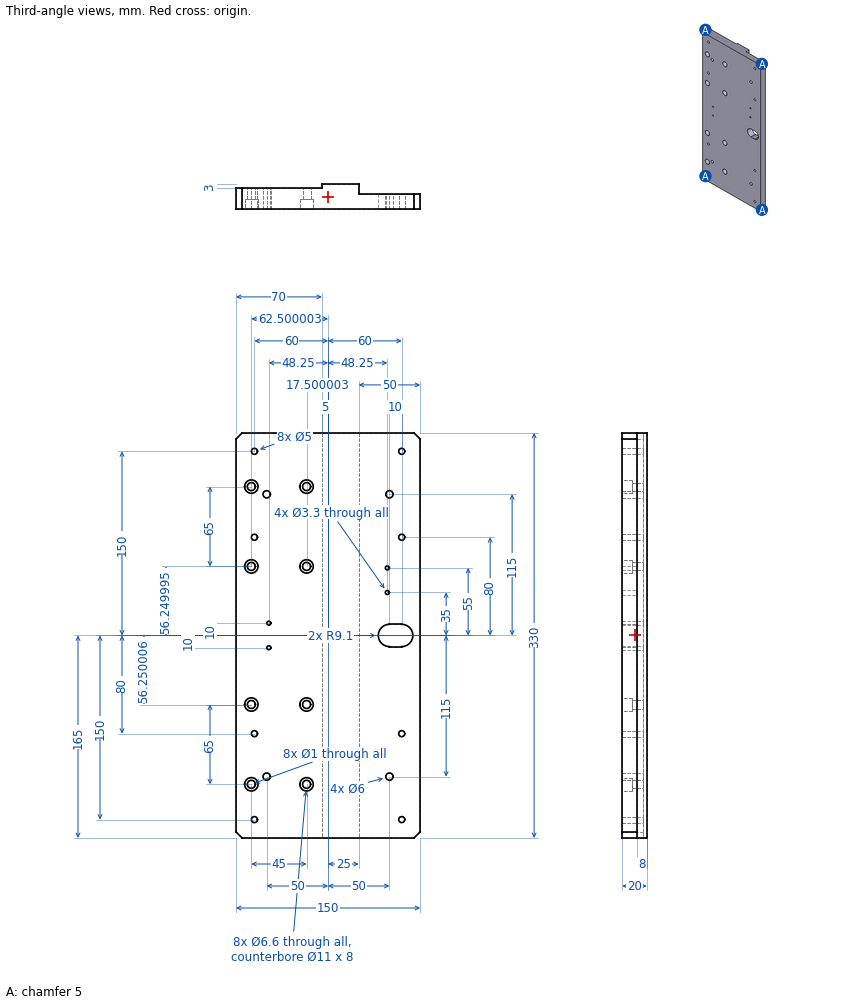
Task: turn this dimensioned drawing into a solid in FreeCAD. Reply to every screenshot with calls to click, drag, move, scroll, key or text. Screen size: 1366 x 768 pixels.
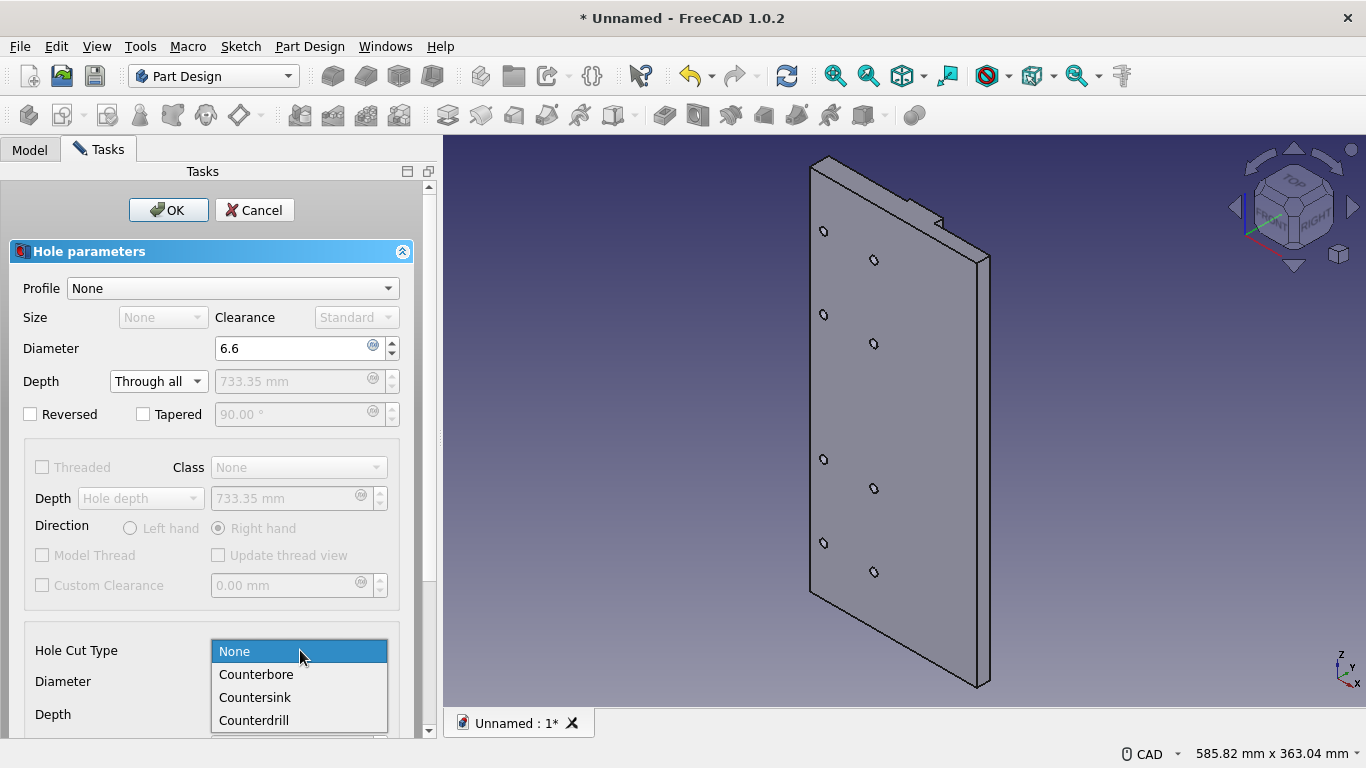
click(298, 674)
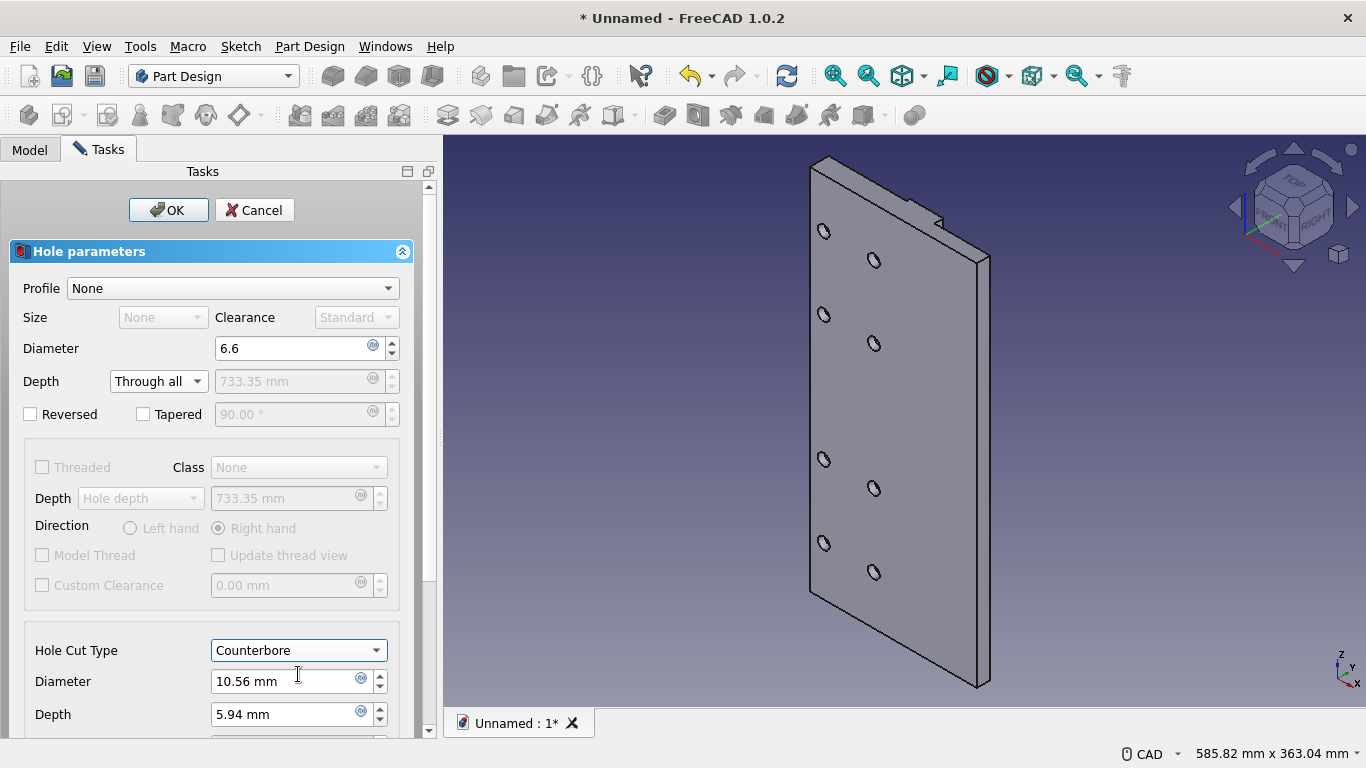
triple_click(292, 682)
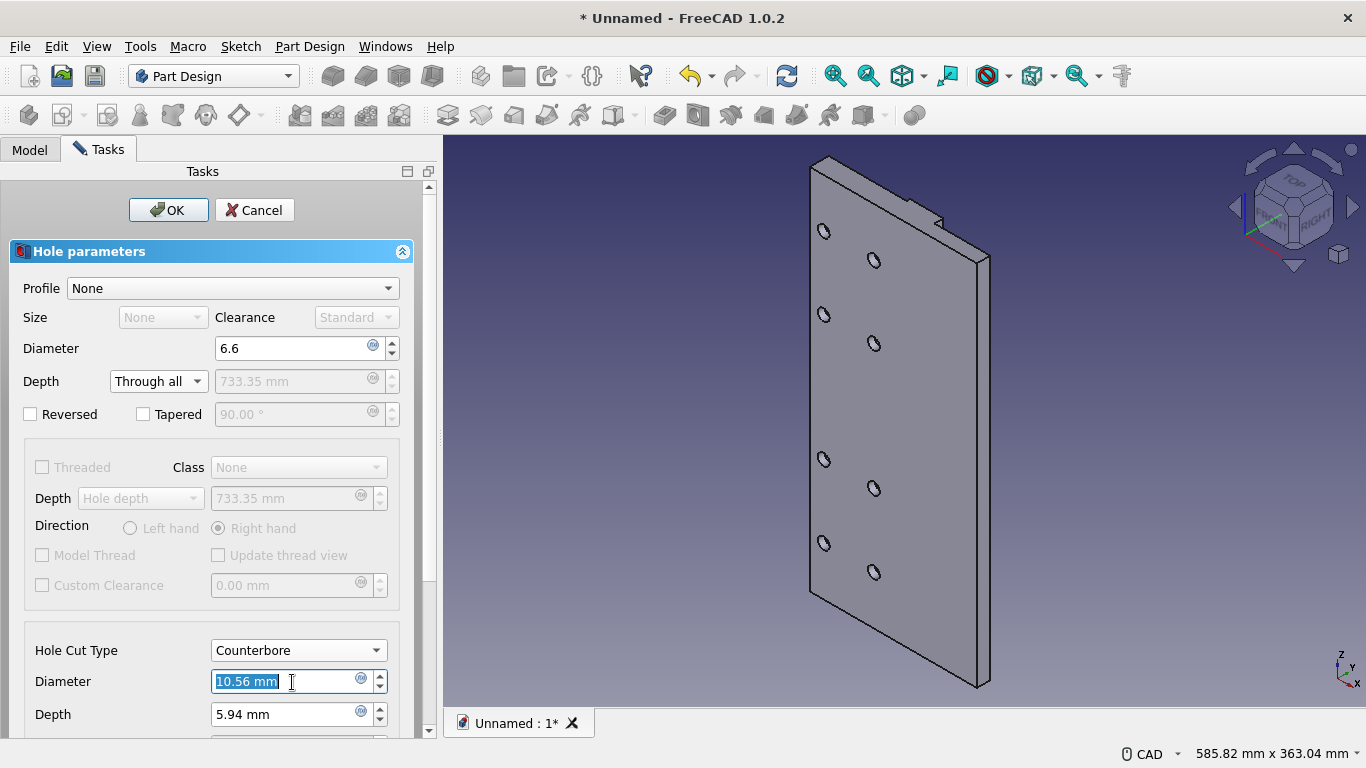
text(11)
key(Tab)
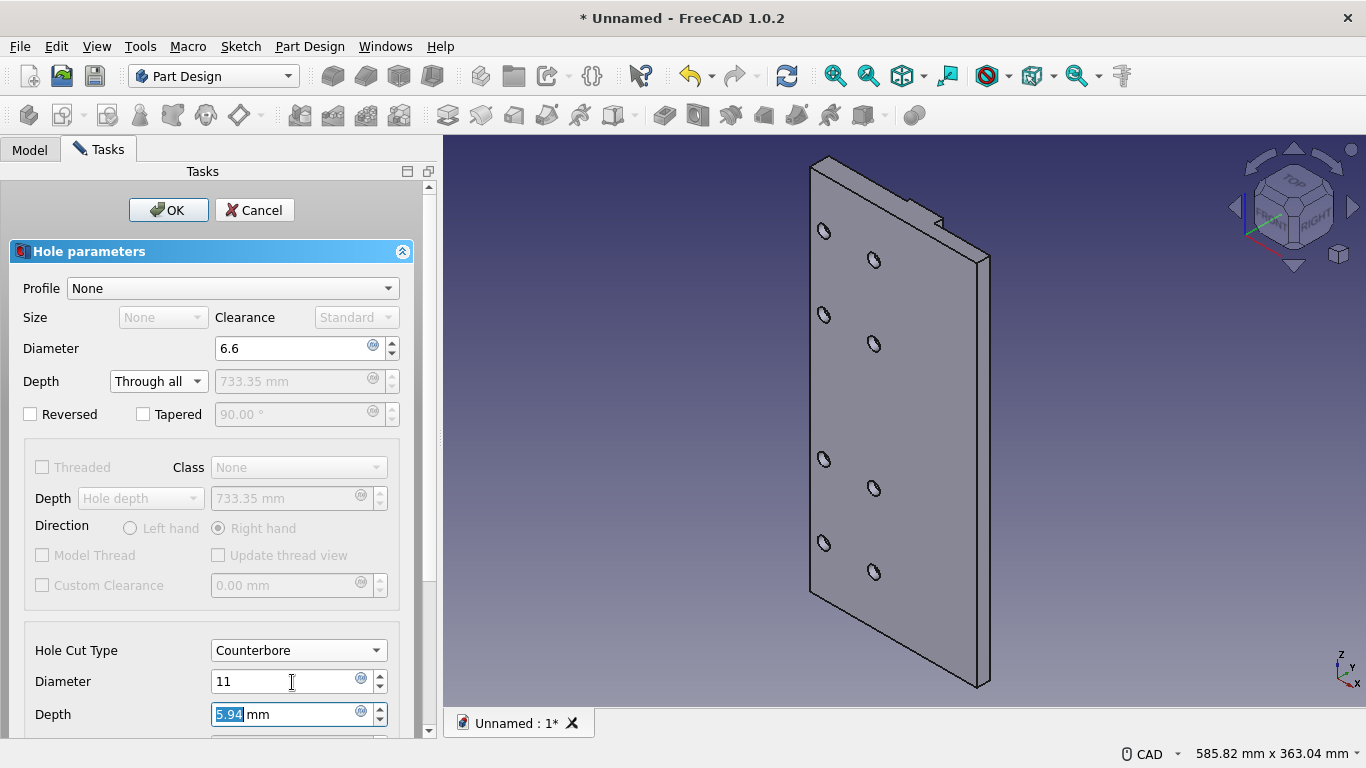
text(8)
key(Tab)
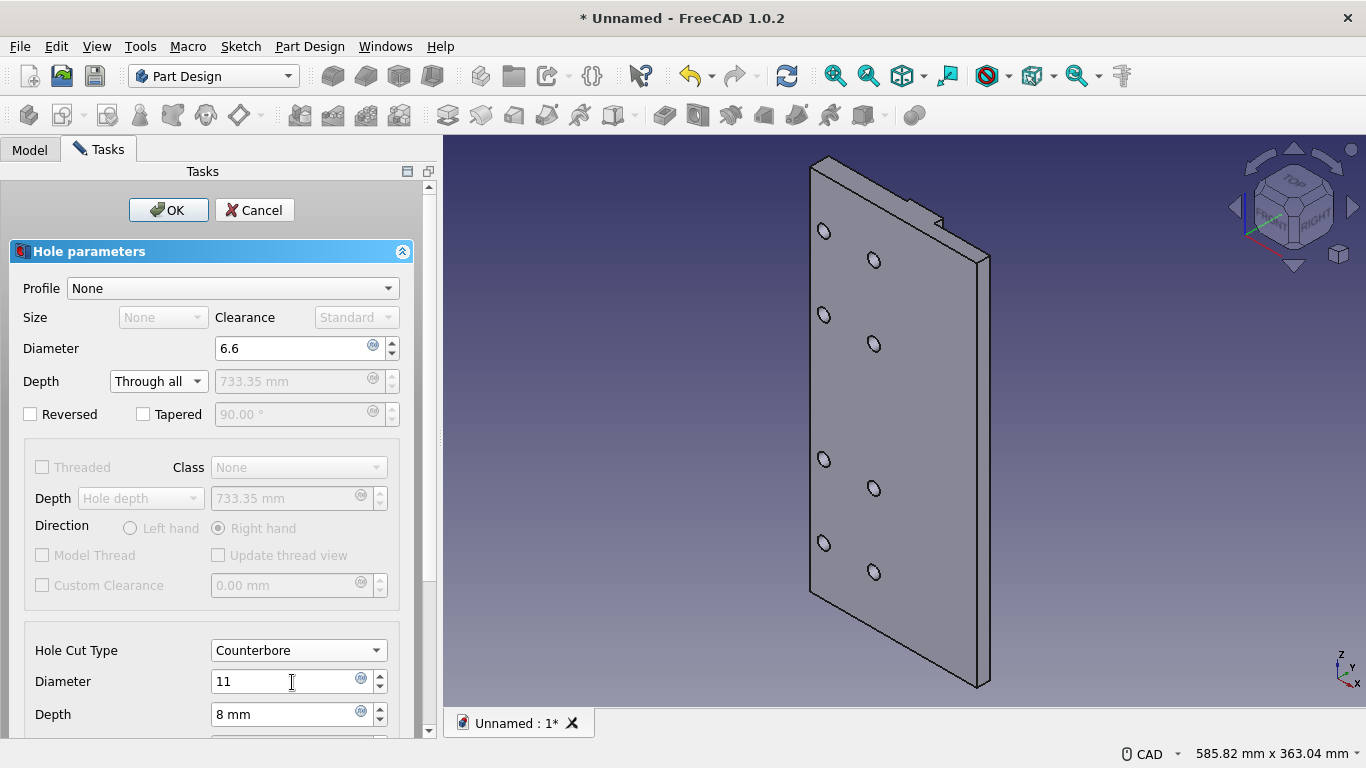
click(169, 210)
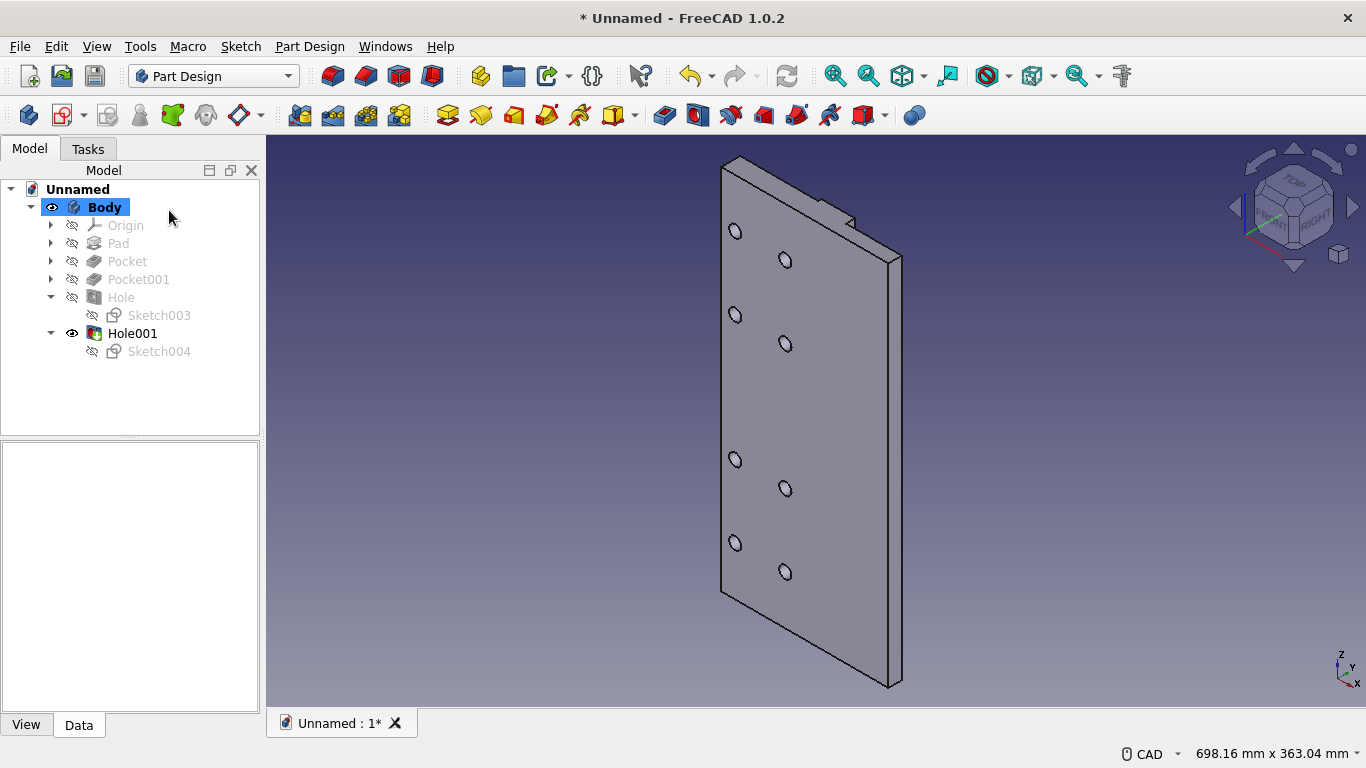
click(829, 440)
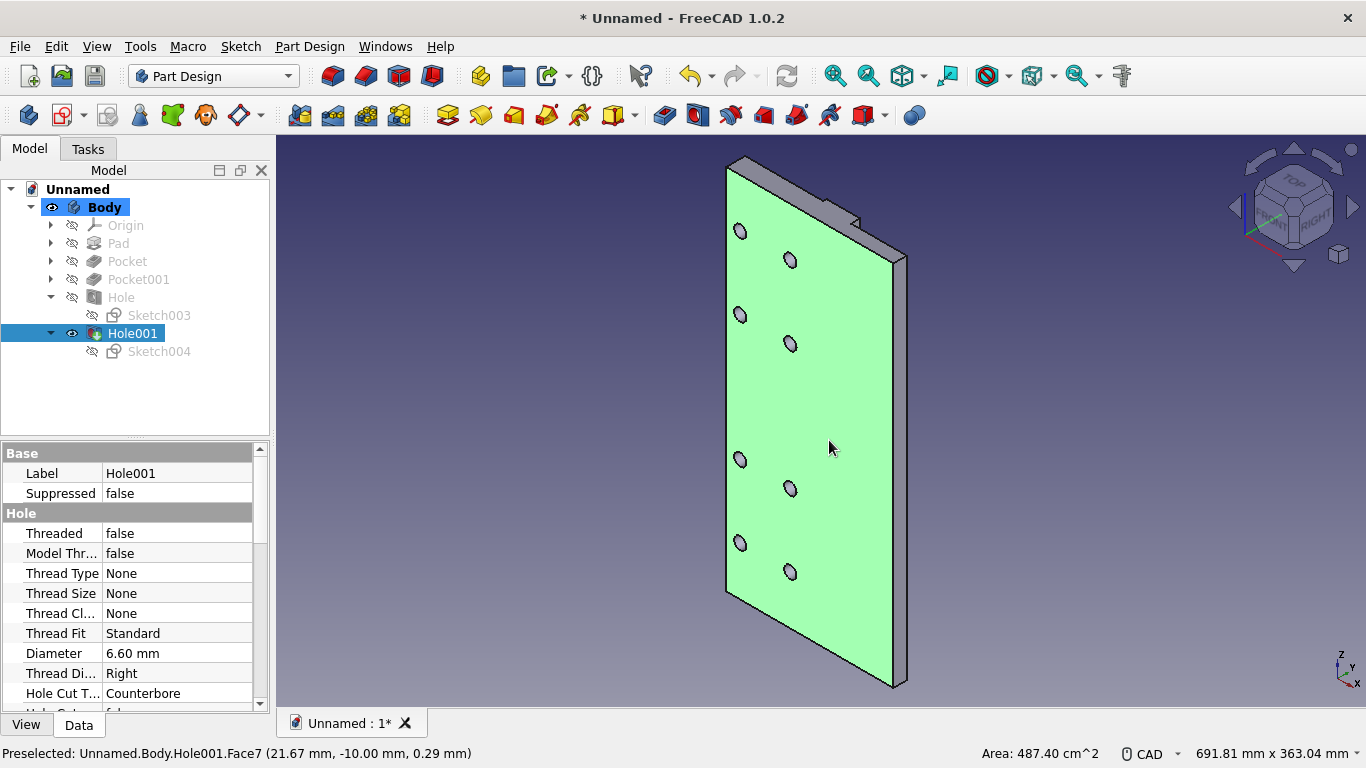
click(62, 116)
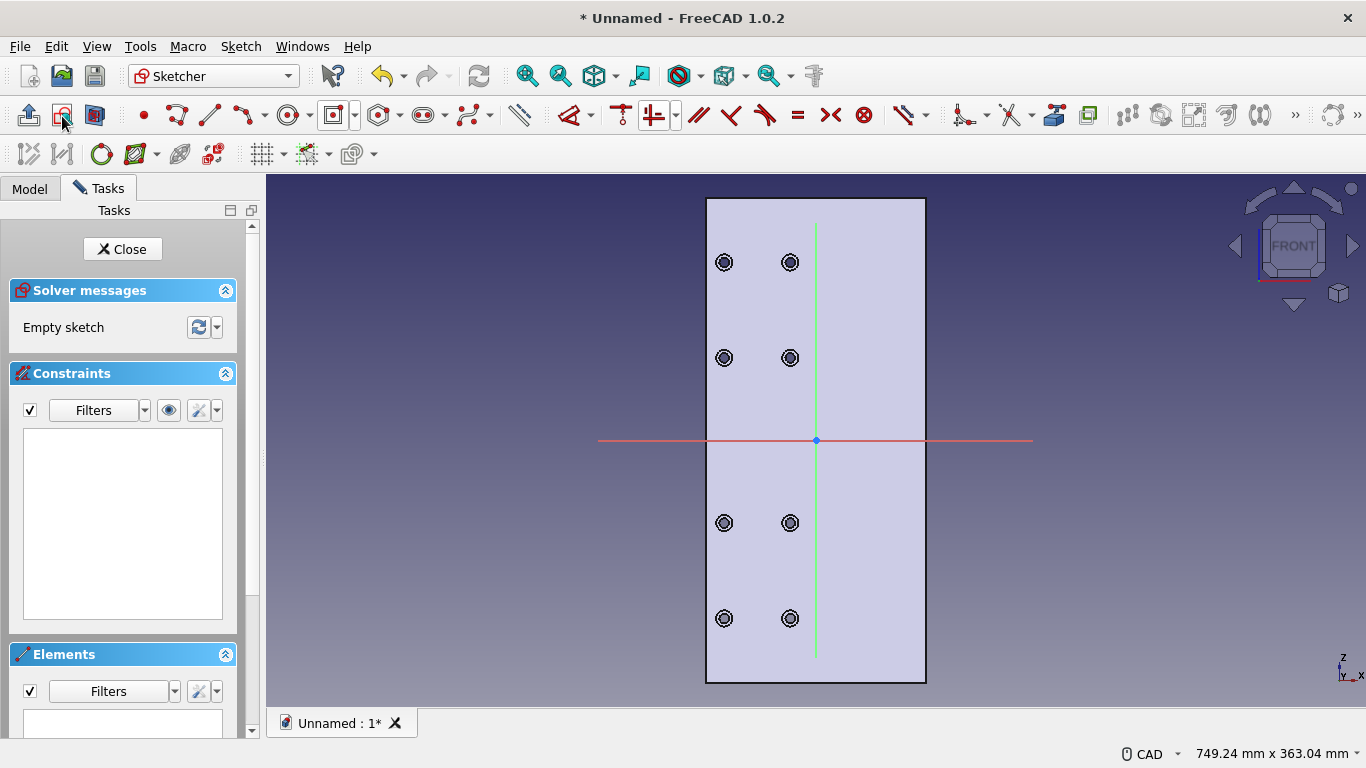
click(288, 116)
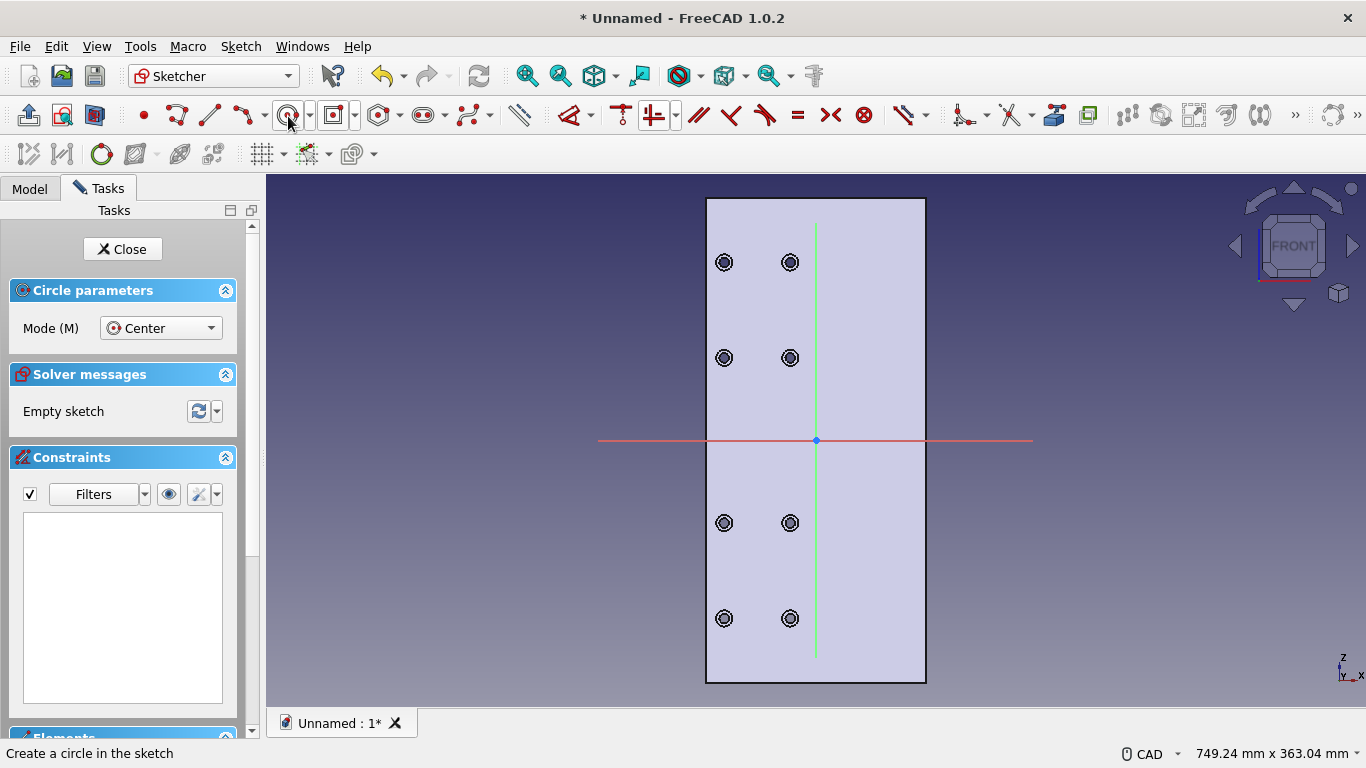
scroll(889, 609, up, 9)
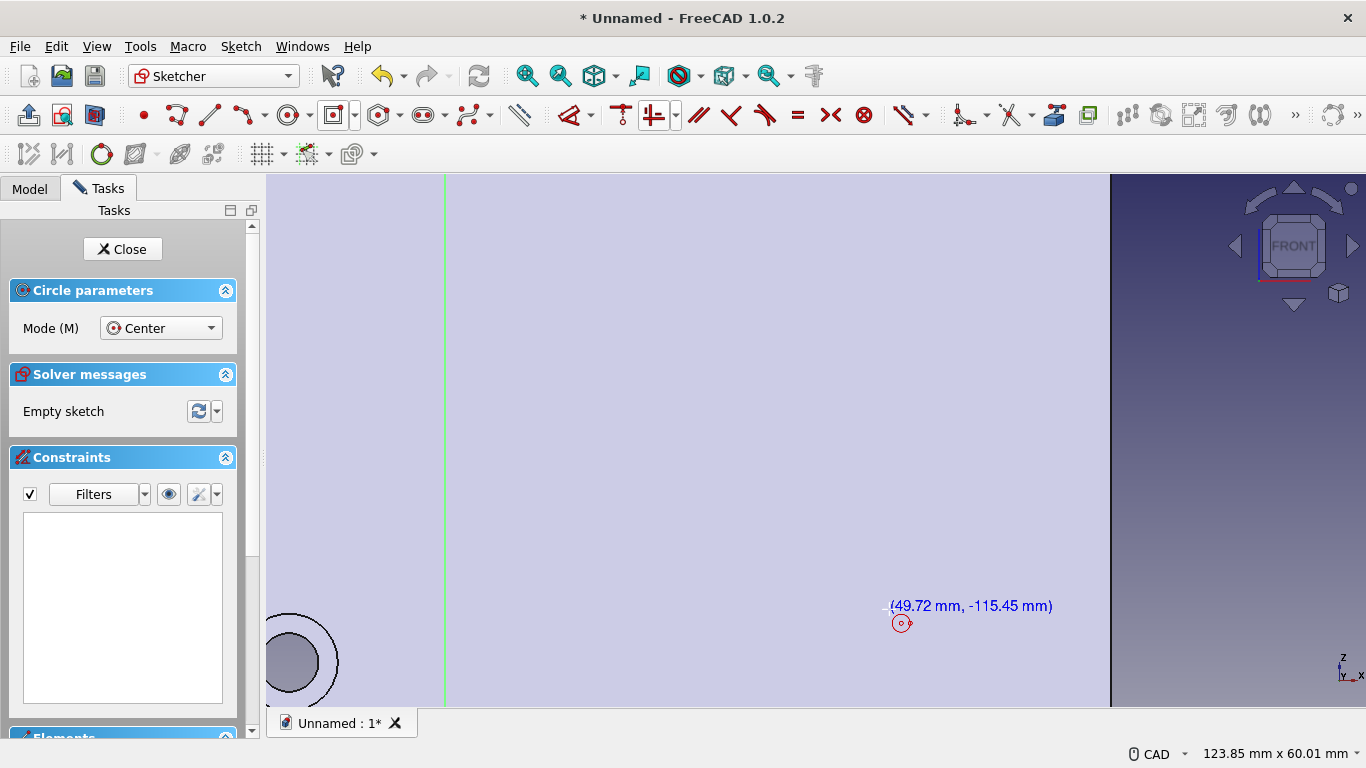
scroll(808, 610, down, 9)